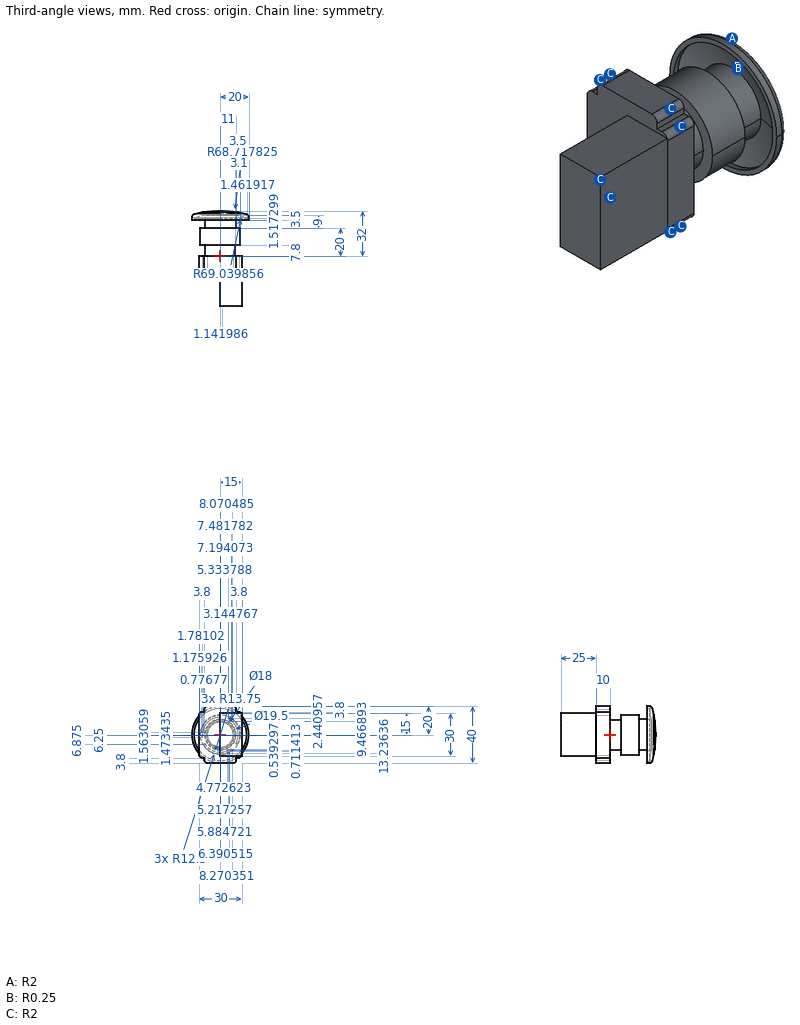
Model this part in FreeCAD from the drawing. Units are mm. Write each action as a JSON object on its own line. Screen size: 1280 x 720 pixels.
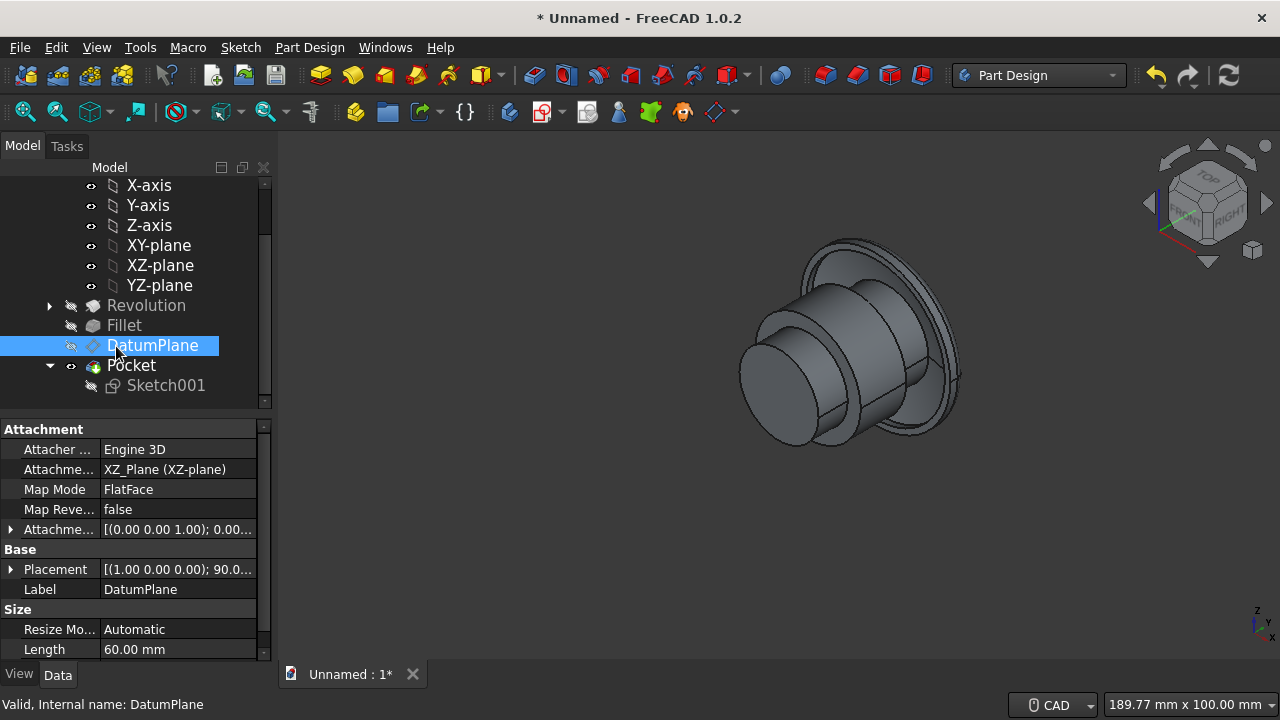
{"action": "key", "text": "4"}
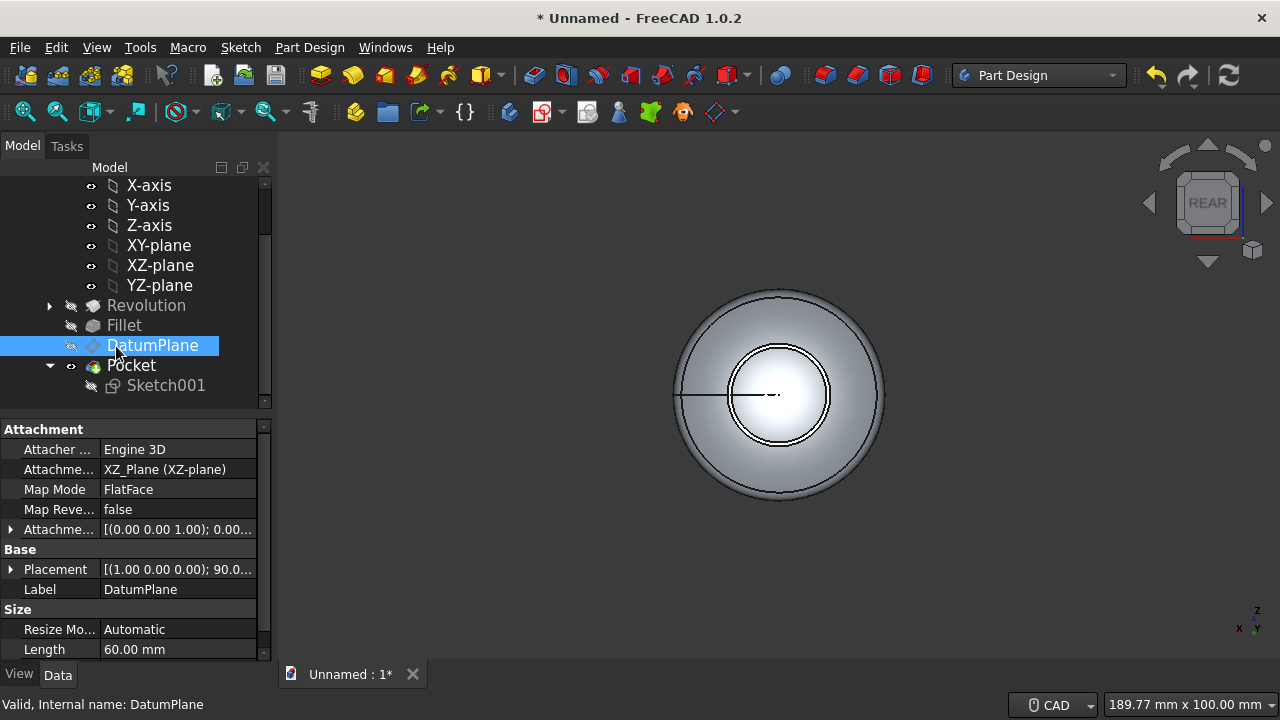
{"action": "left_click", "coordinate": [26, 112]}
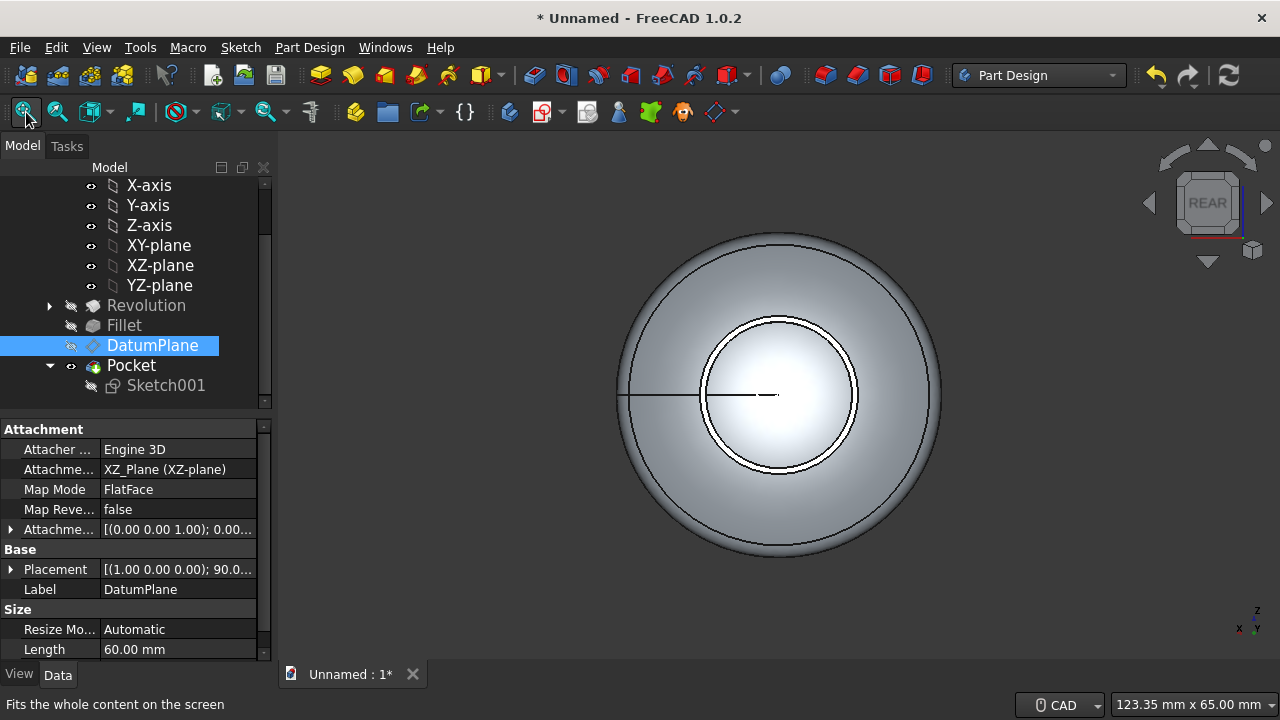
{"action": "scroll", "coordinate": [743, 326], "scroll_direction": "up", "scroll_amount": 9}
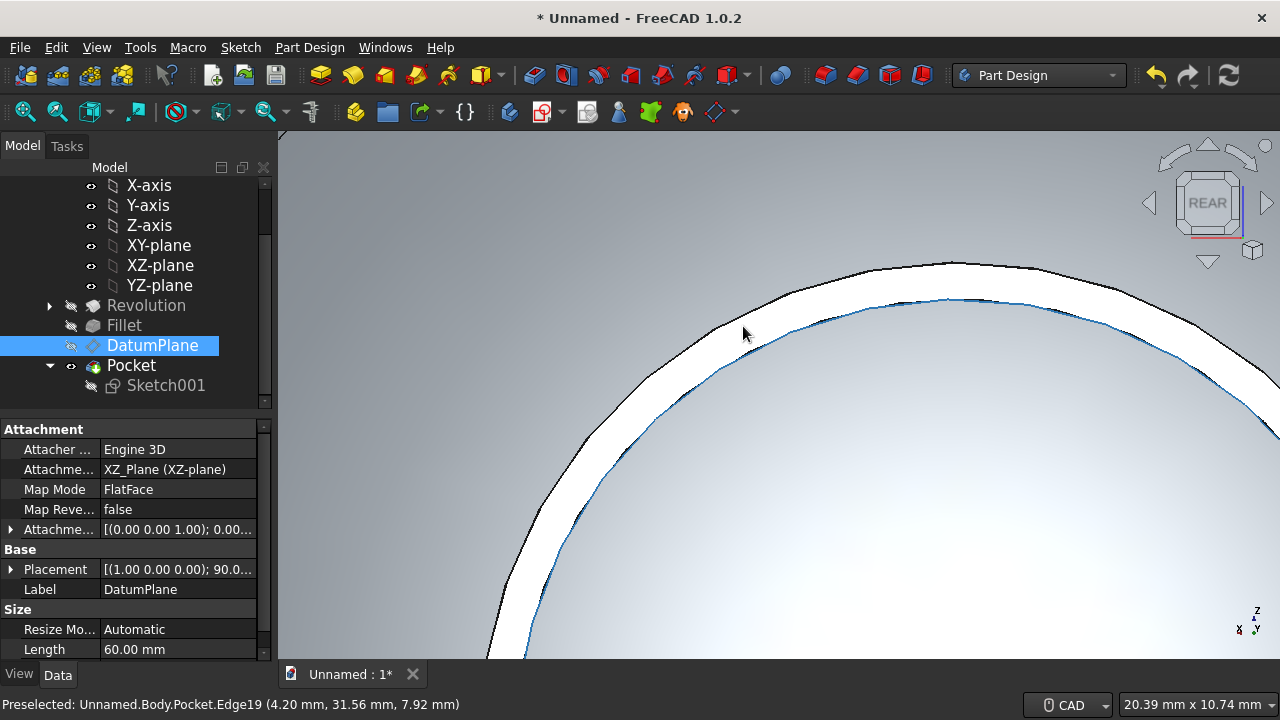
{"action": "left_click", "coordinate": [738, 329]}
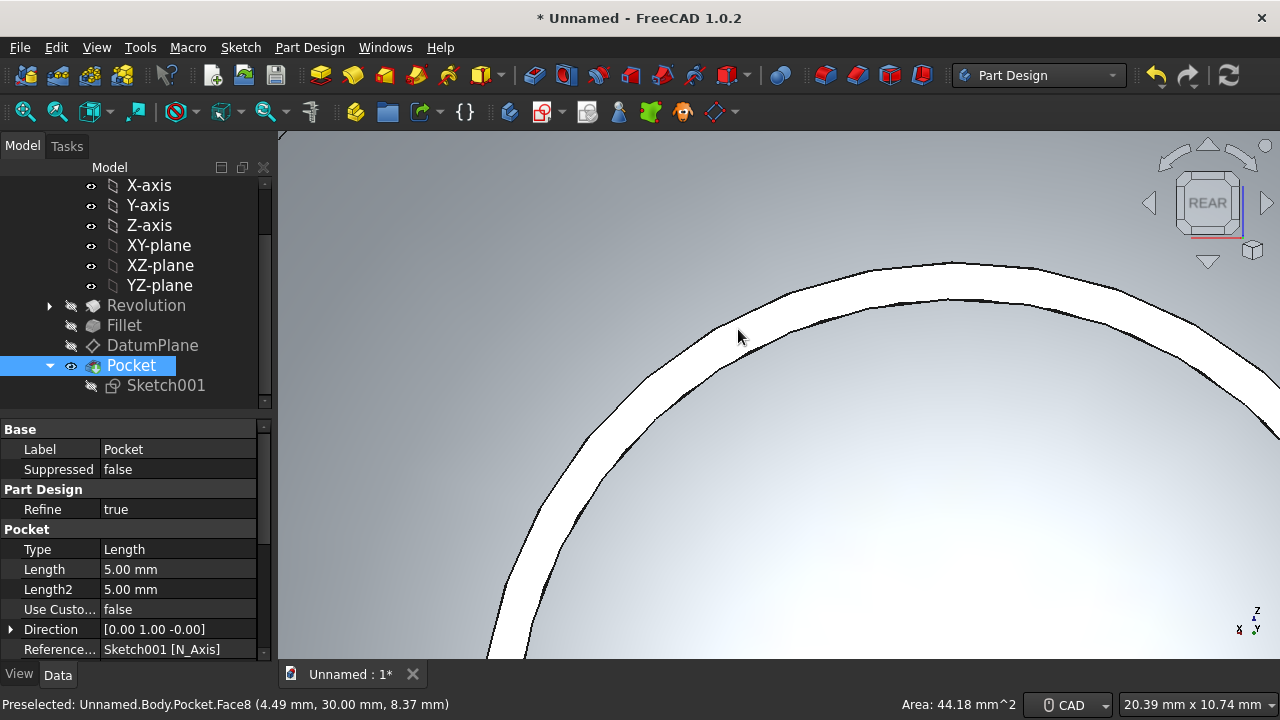
{"action": "left_click", "coordinate": [542, 112]}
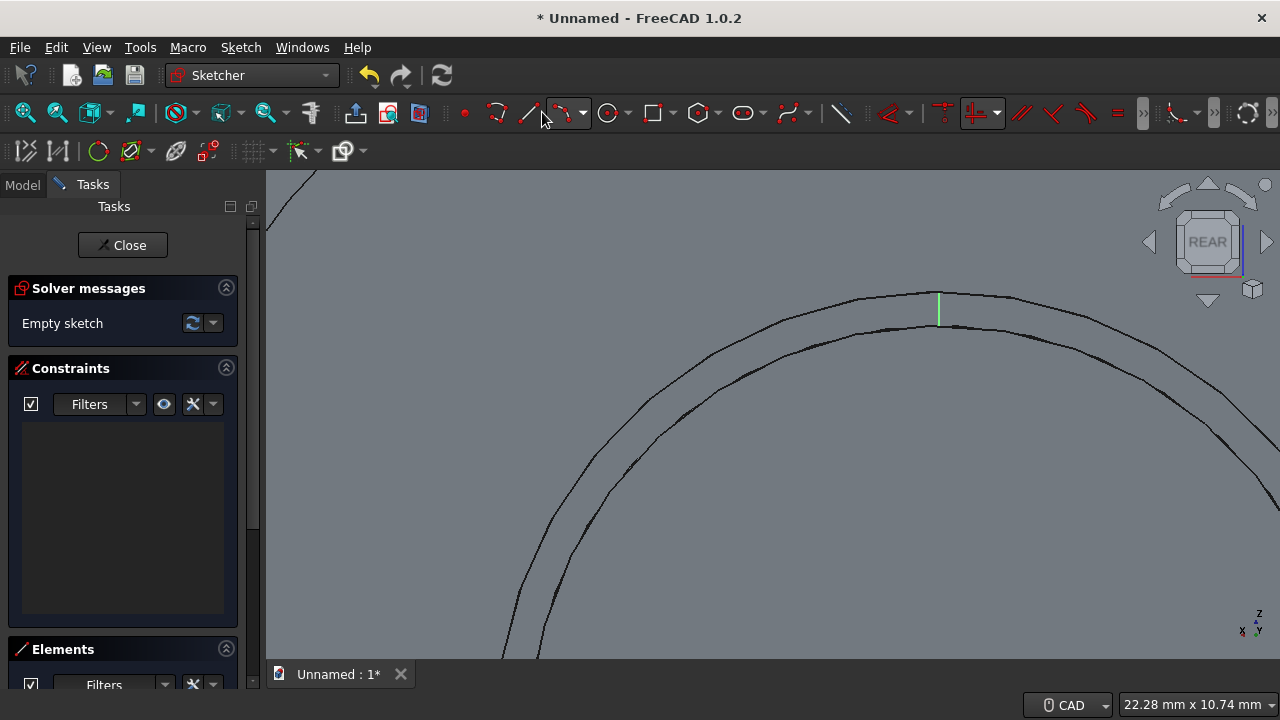
{"action": "scroll", "coordinate": [617, 313], "scroll_direction": "down", "scroll_amount": 7}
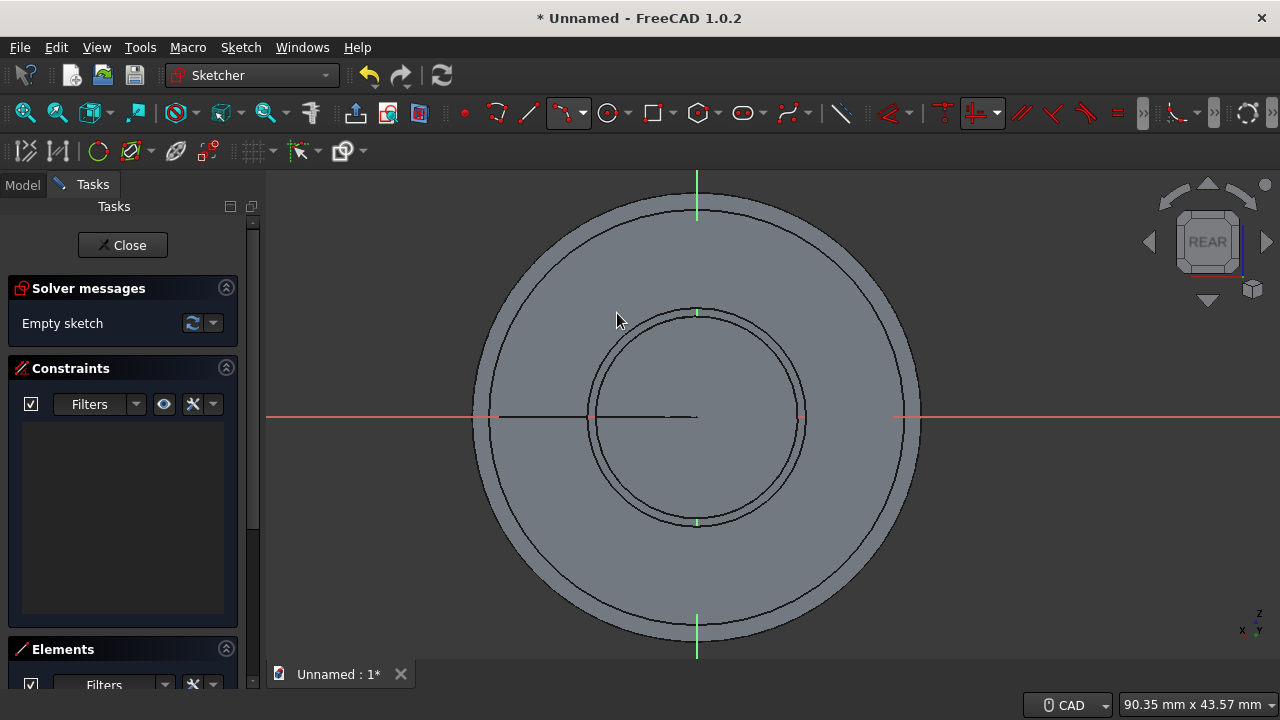
{"action": "left_click", "coordinate": [530, 114]}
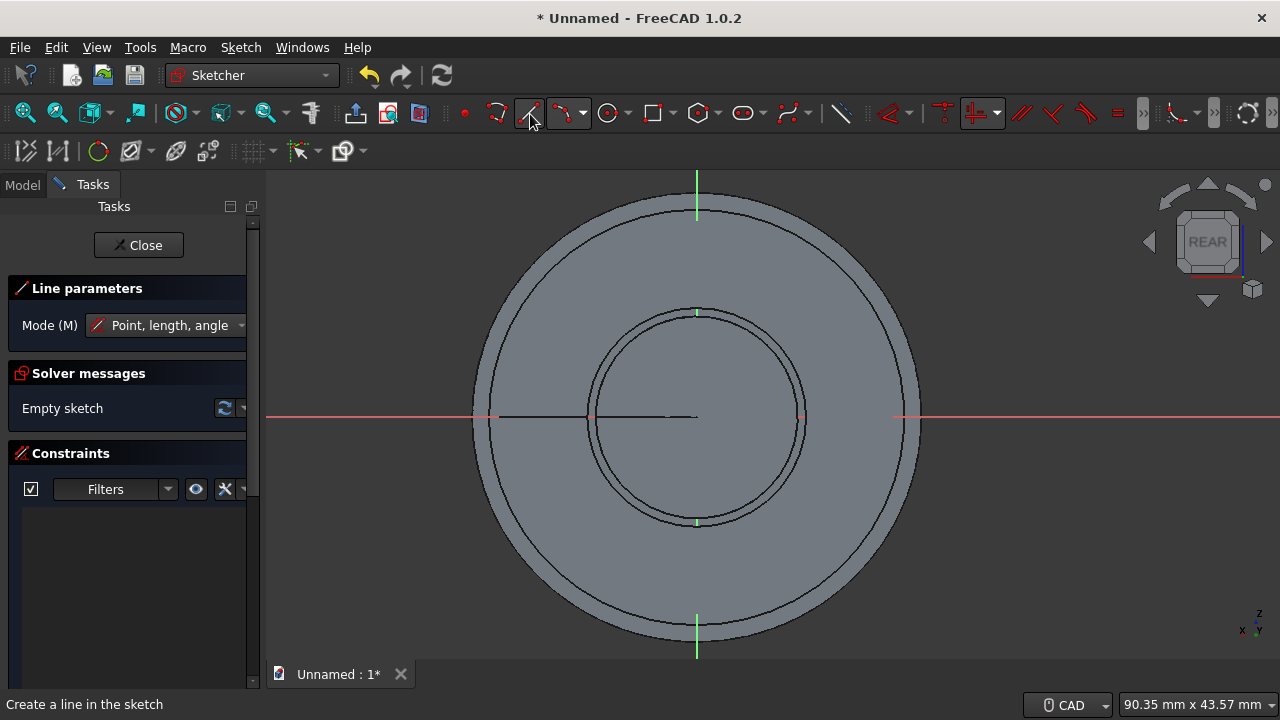
{"action": "left_click", "coordinate": [830, 495]}
{"action": "left_click", "coordinate": [818, 488]}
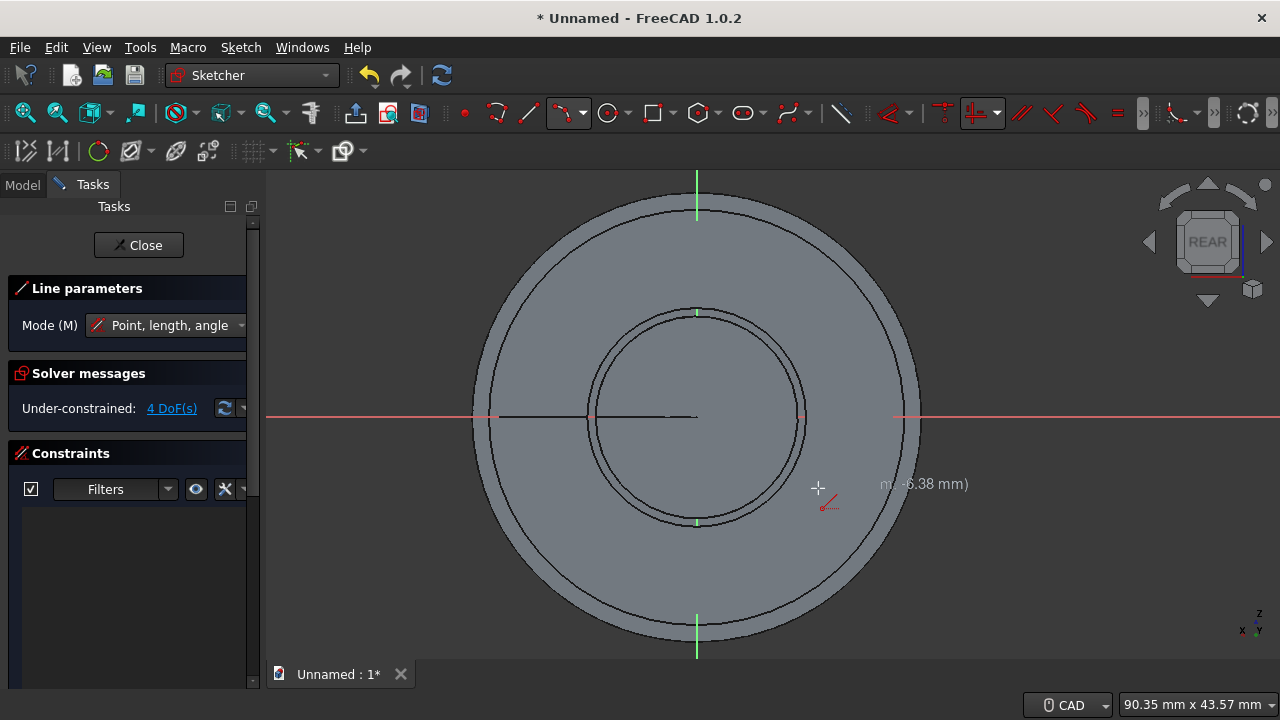
{"action": "left_click", "coordinate": [498, 114]}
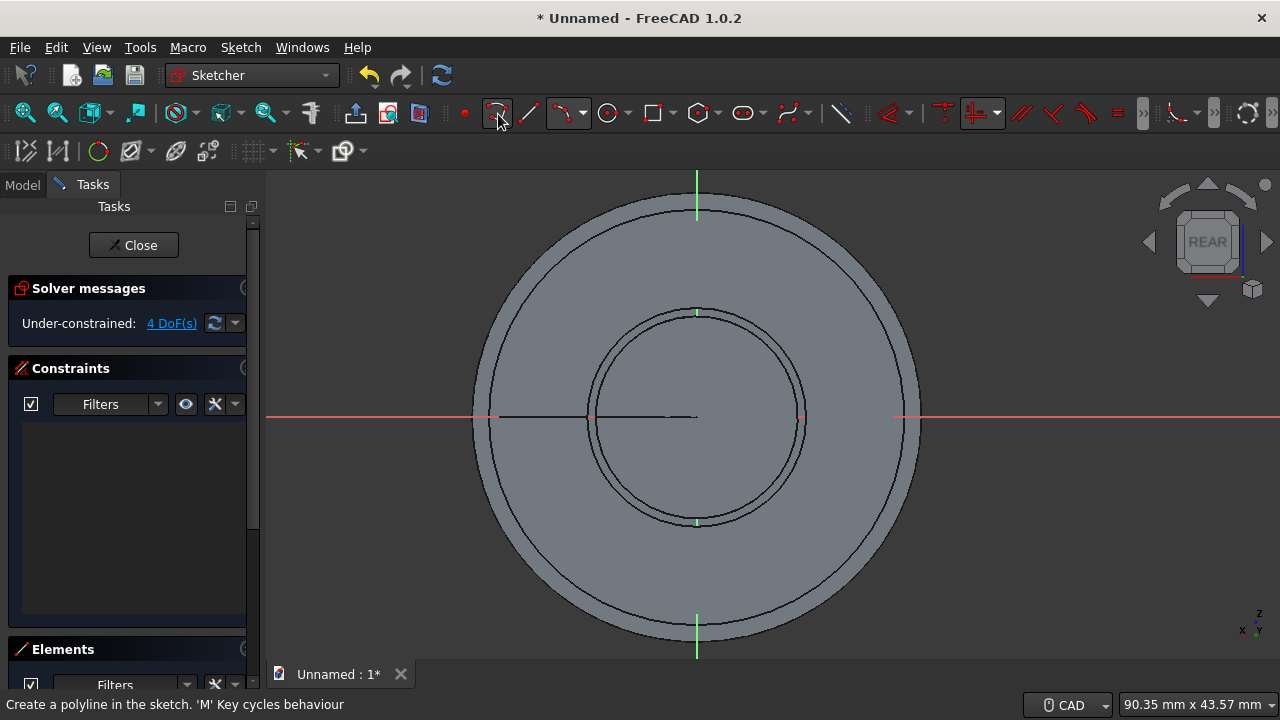
{"action": "left_click", "coordinate": [638, 545]}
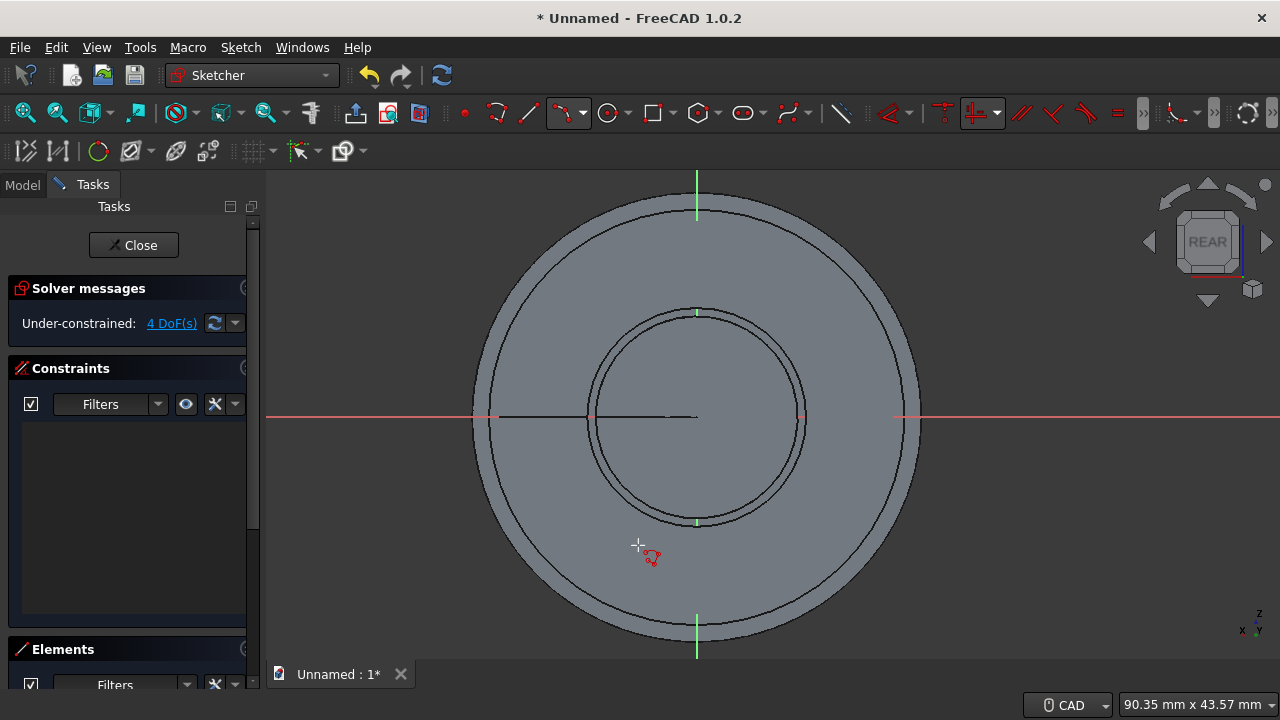
{"action": "scroll", "coordinate": [643, 537], "scroll_direction": "up", "scroll_amount": 3}